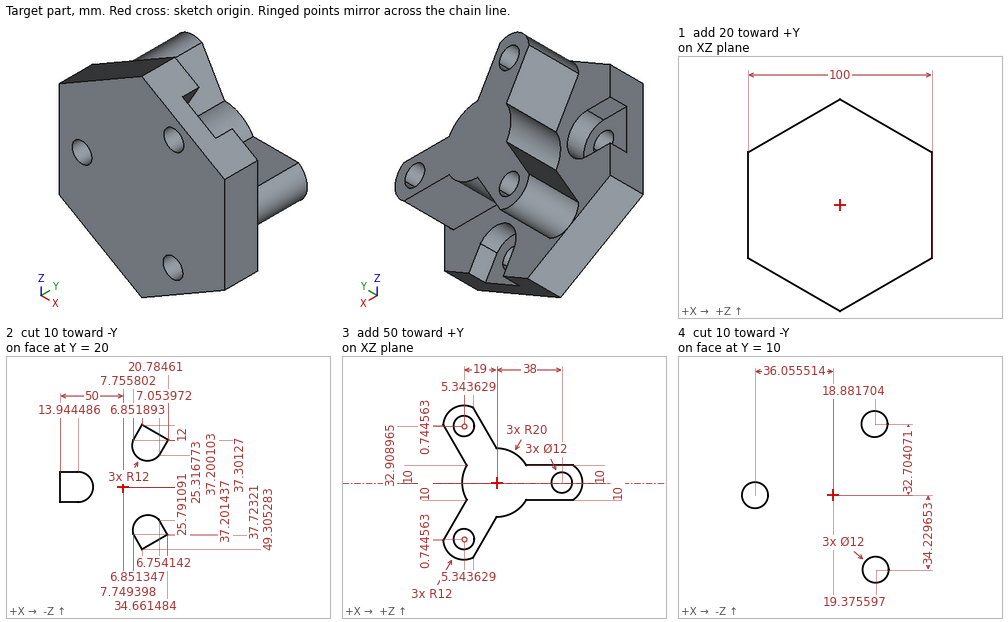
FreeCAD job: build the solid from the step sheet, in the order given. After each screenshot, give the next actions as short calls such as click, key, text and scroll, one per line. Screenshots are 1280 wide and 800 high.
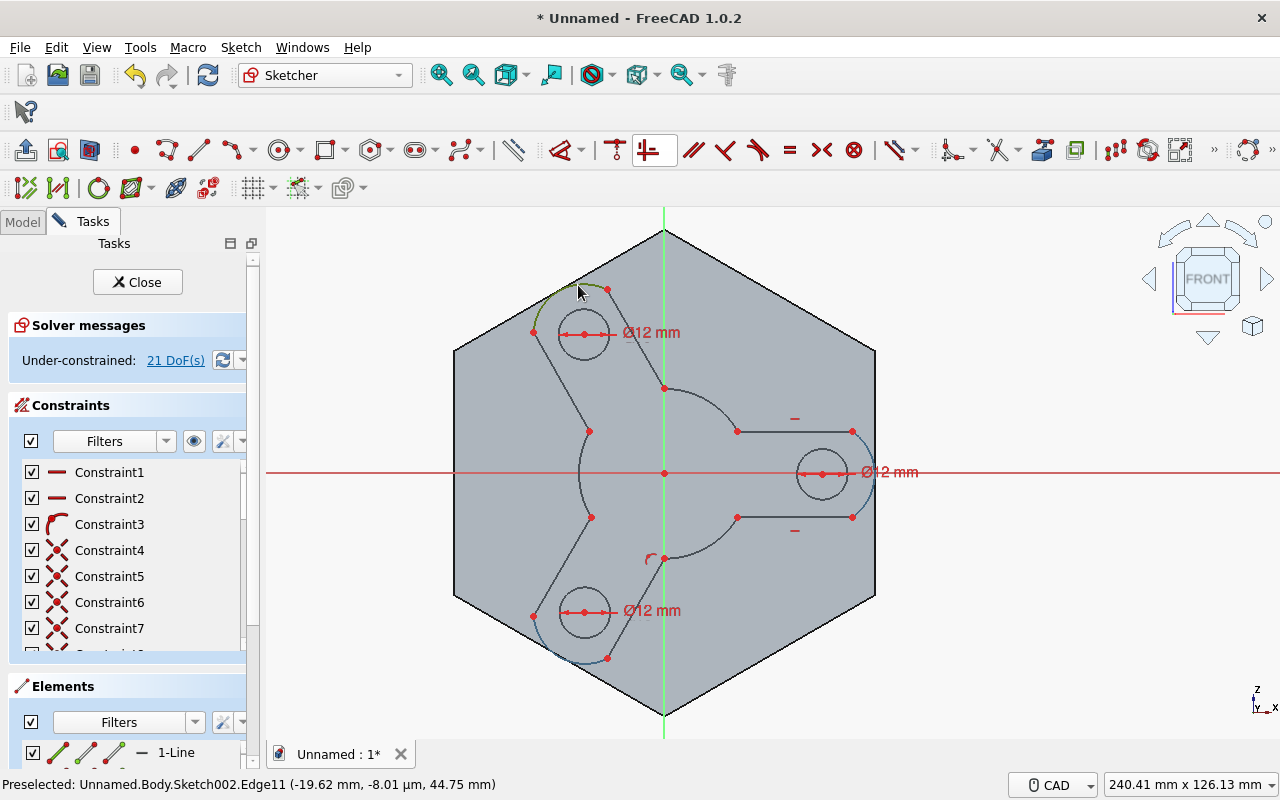
click(790, 150)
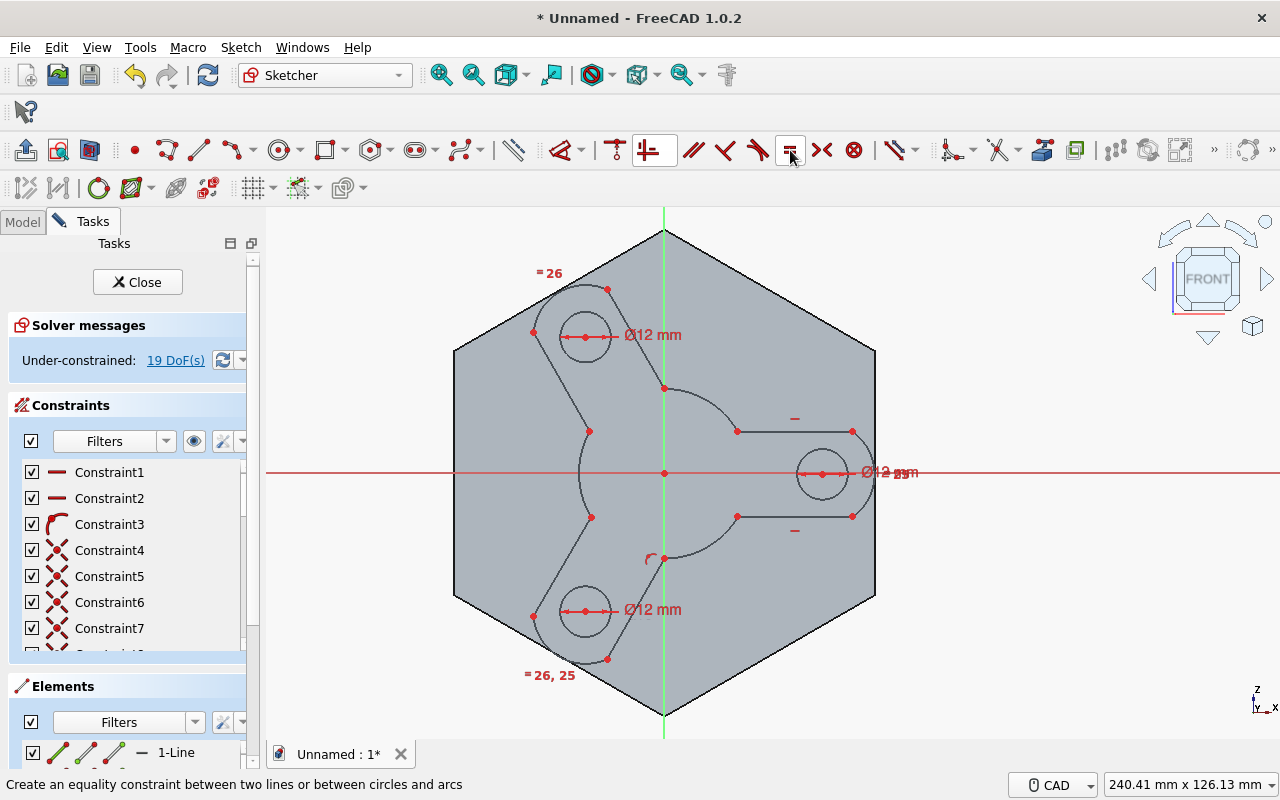
click(691, 555)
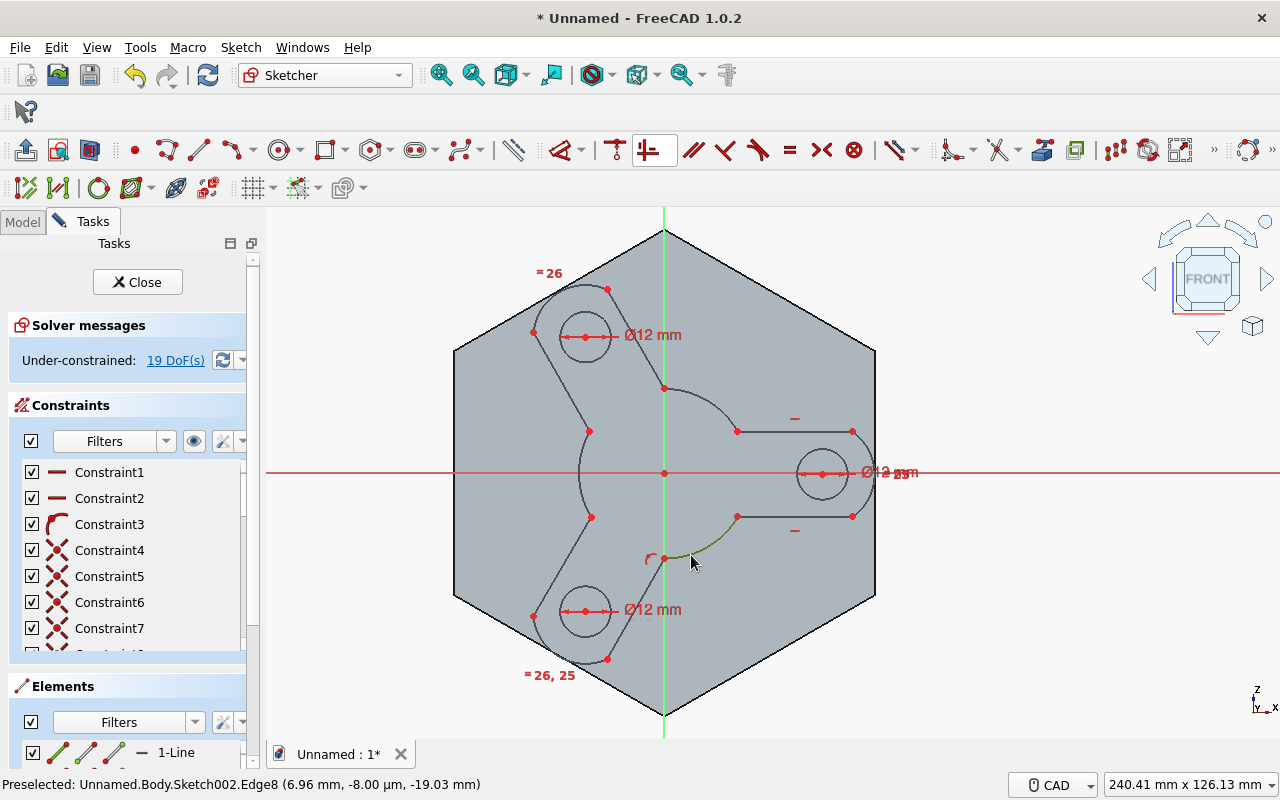
click(581, 457)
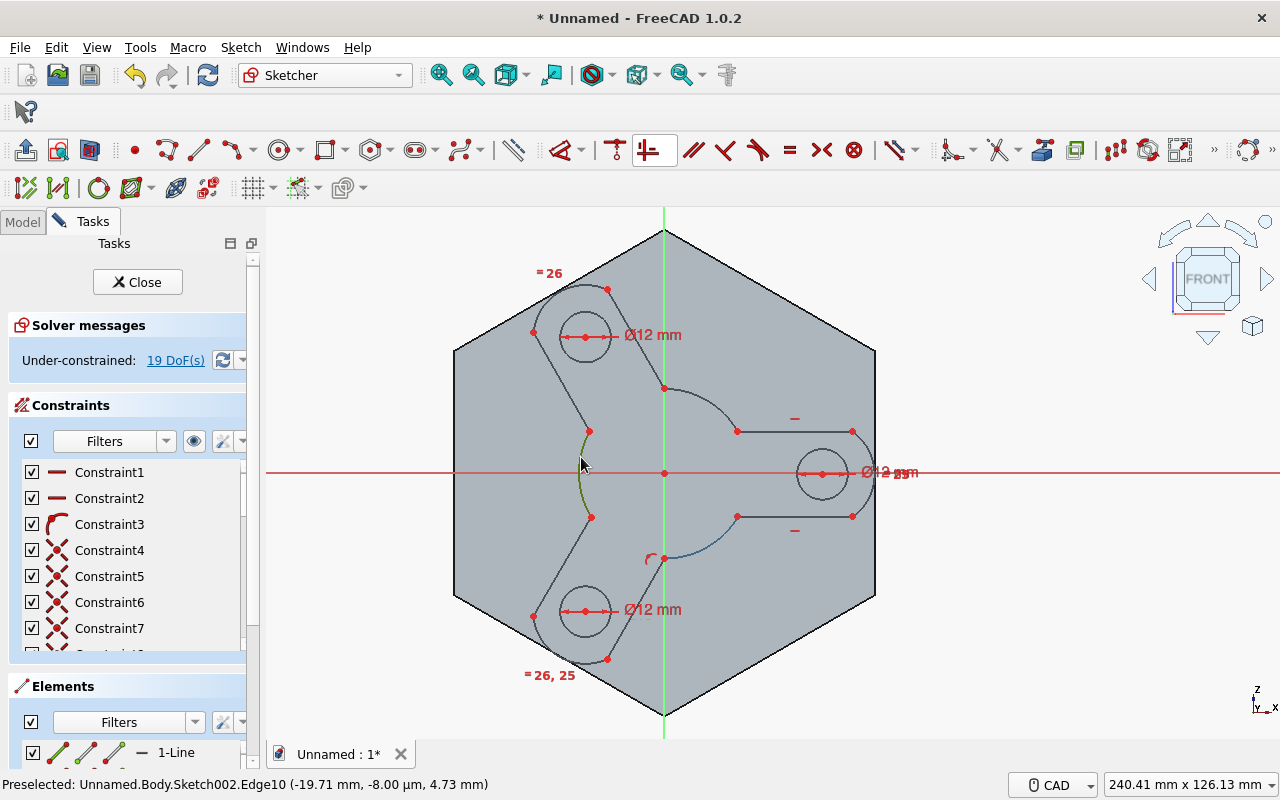
click(721, 411)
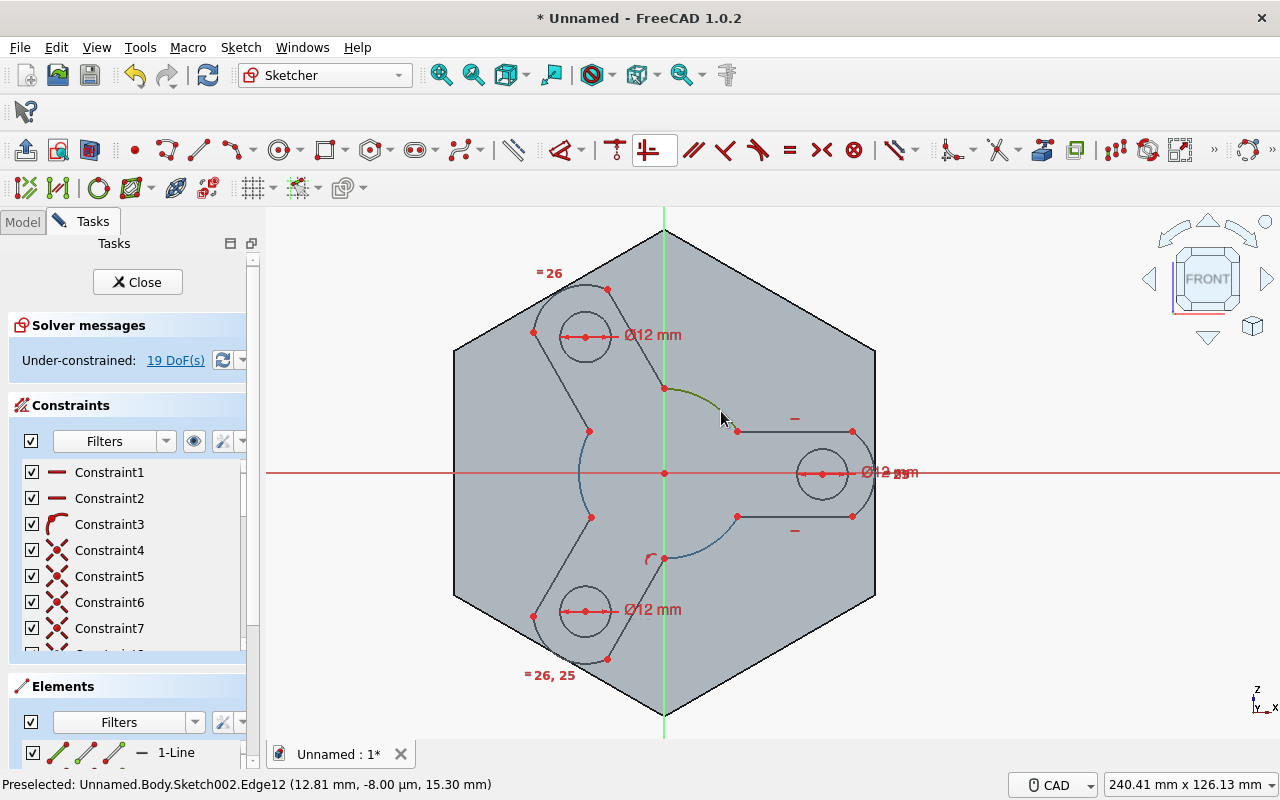
click(790, 150)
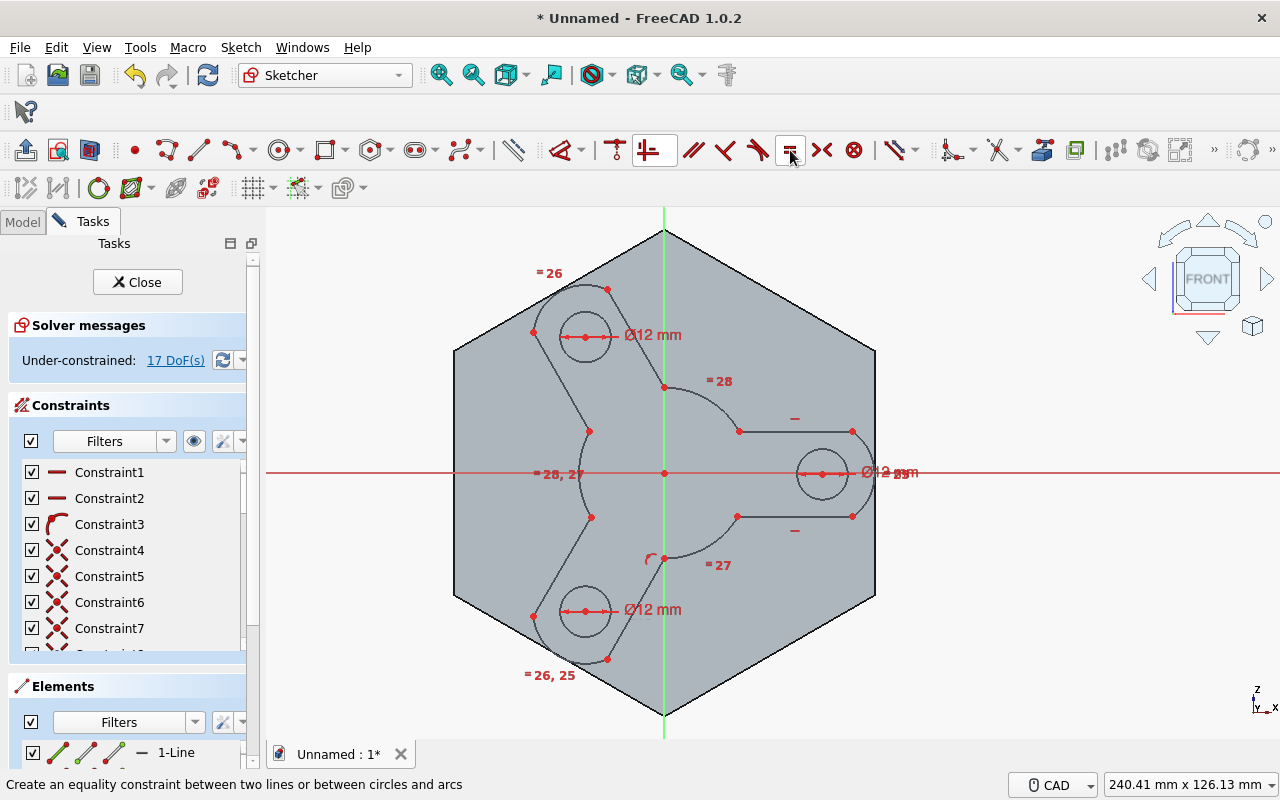
click(822, 474)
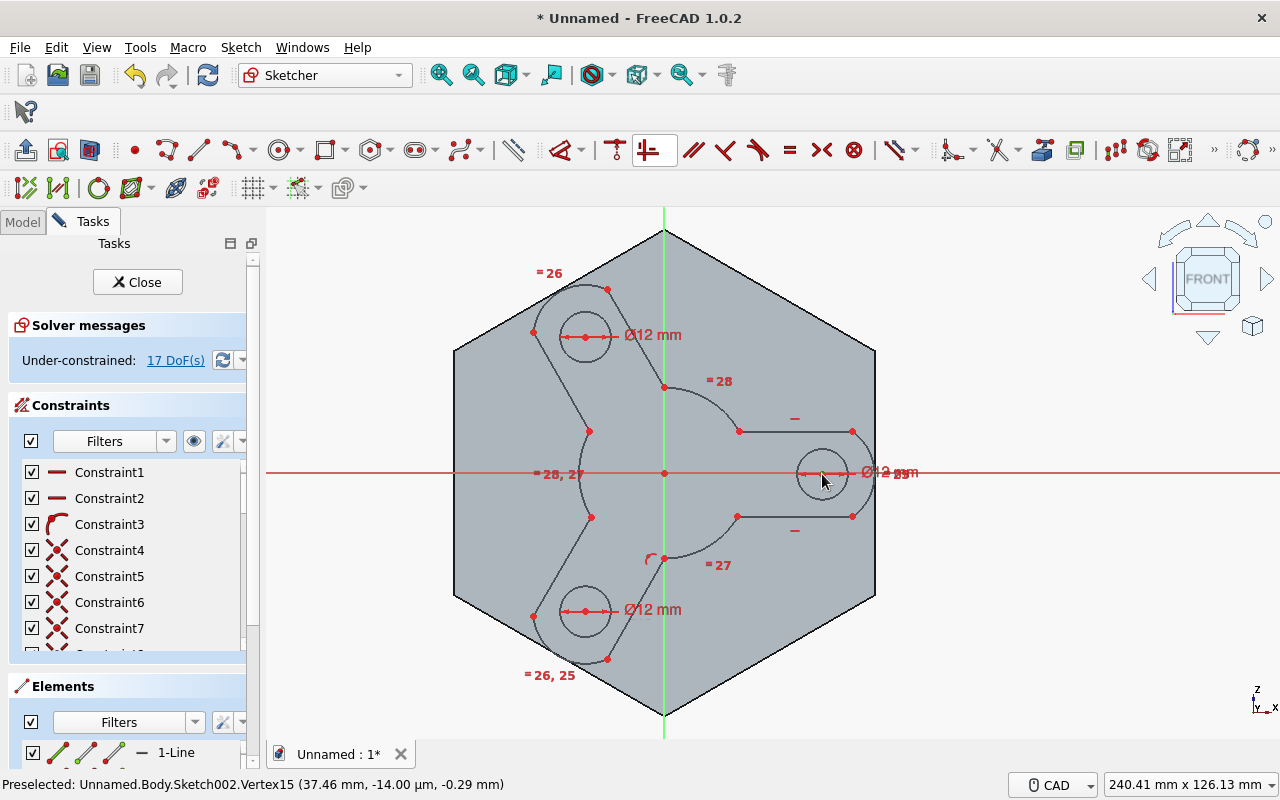
click(353, 473)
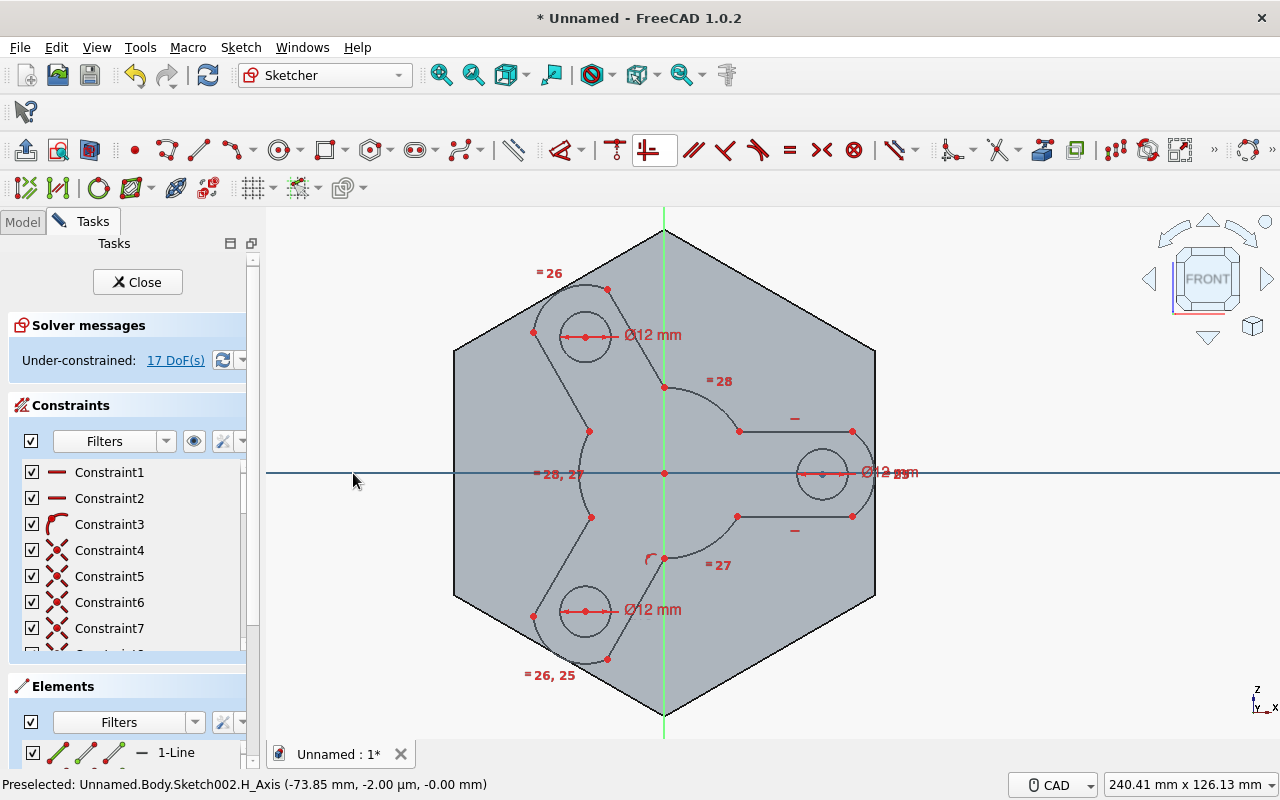
key(c)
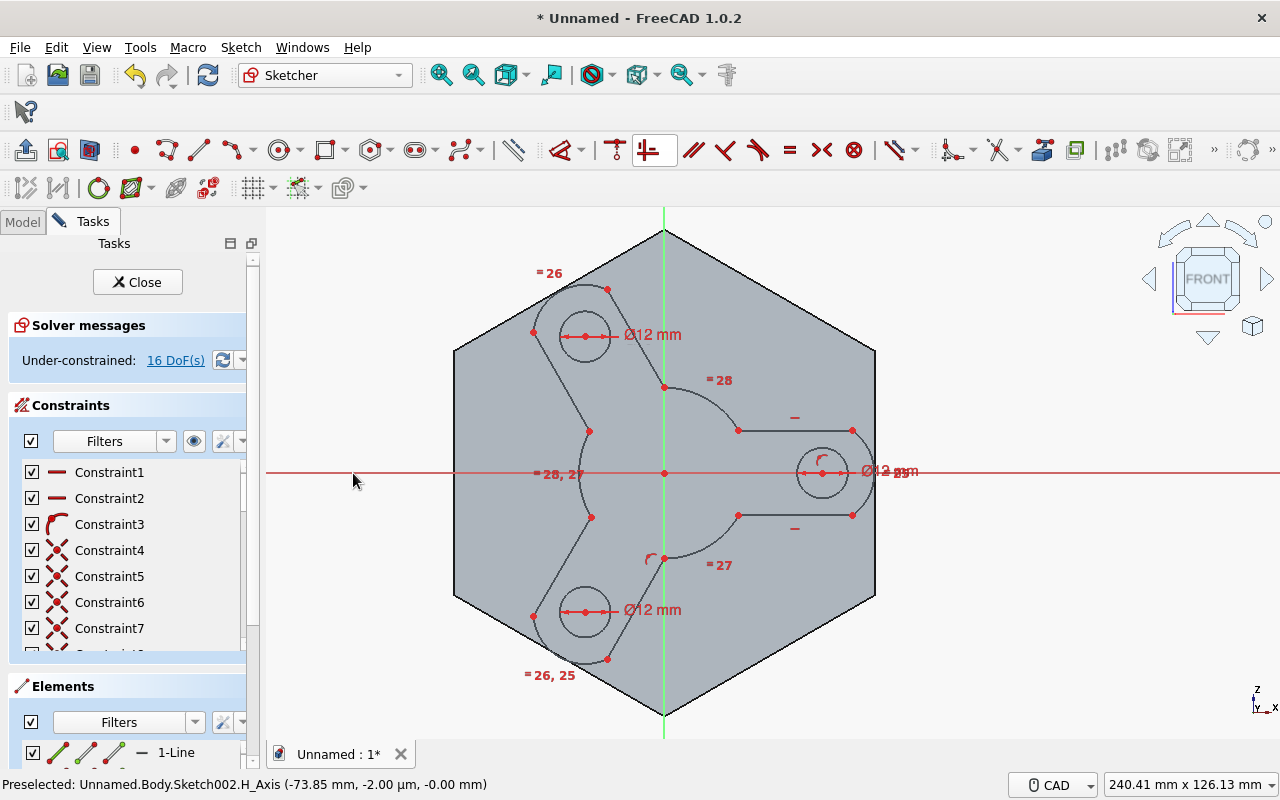
click(585, 612)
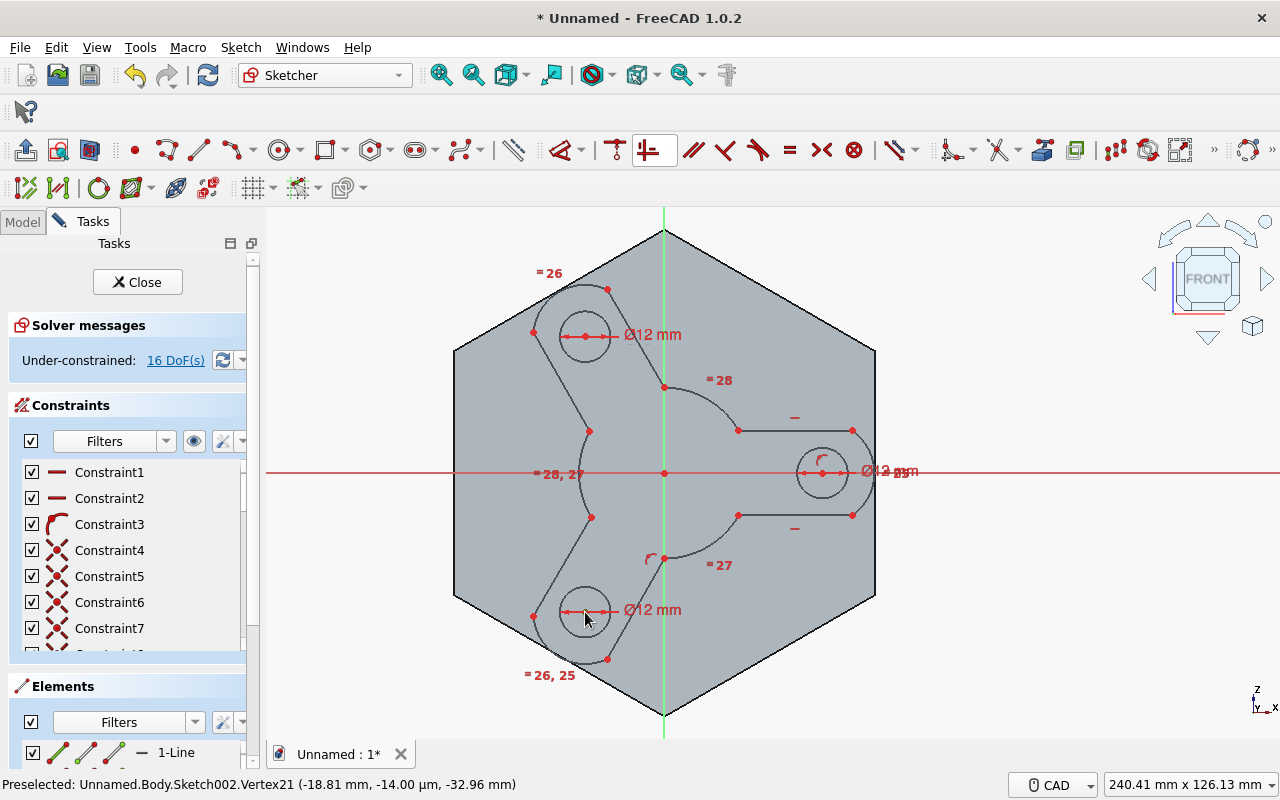
click(585, 337)